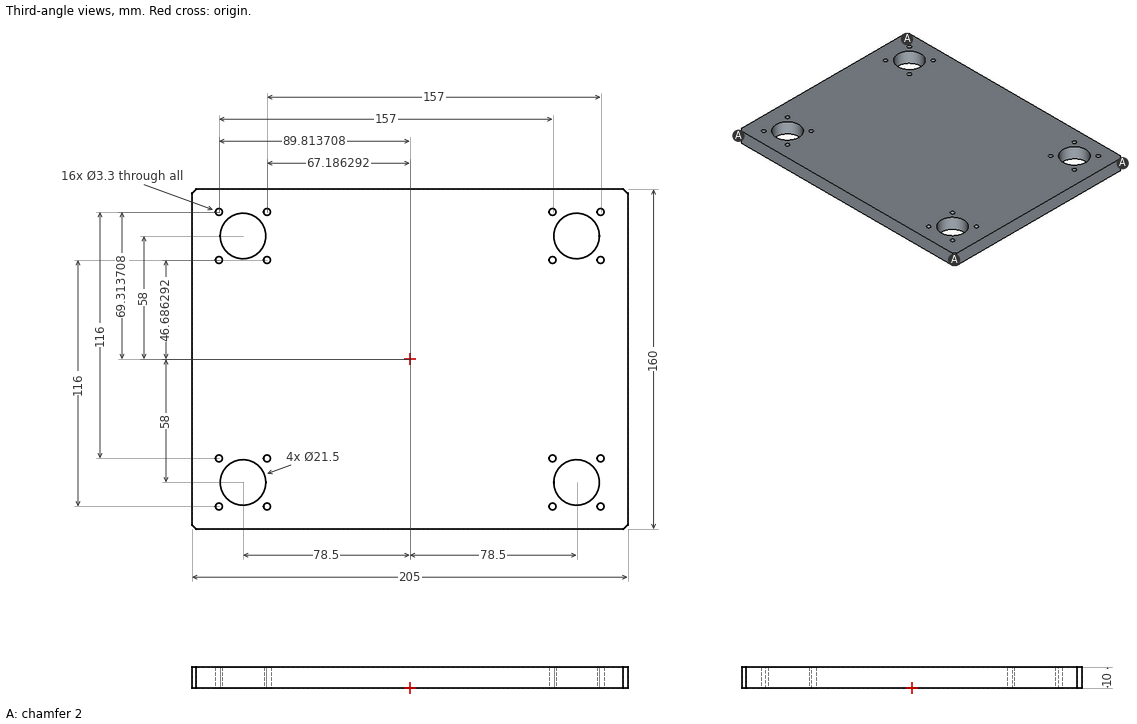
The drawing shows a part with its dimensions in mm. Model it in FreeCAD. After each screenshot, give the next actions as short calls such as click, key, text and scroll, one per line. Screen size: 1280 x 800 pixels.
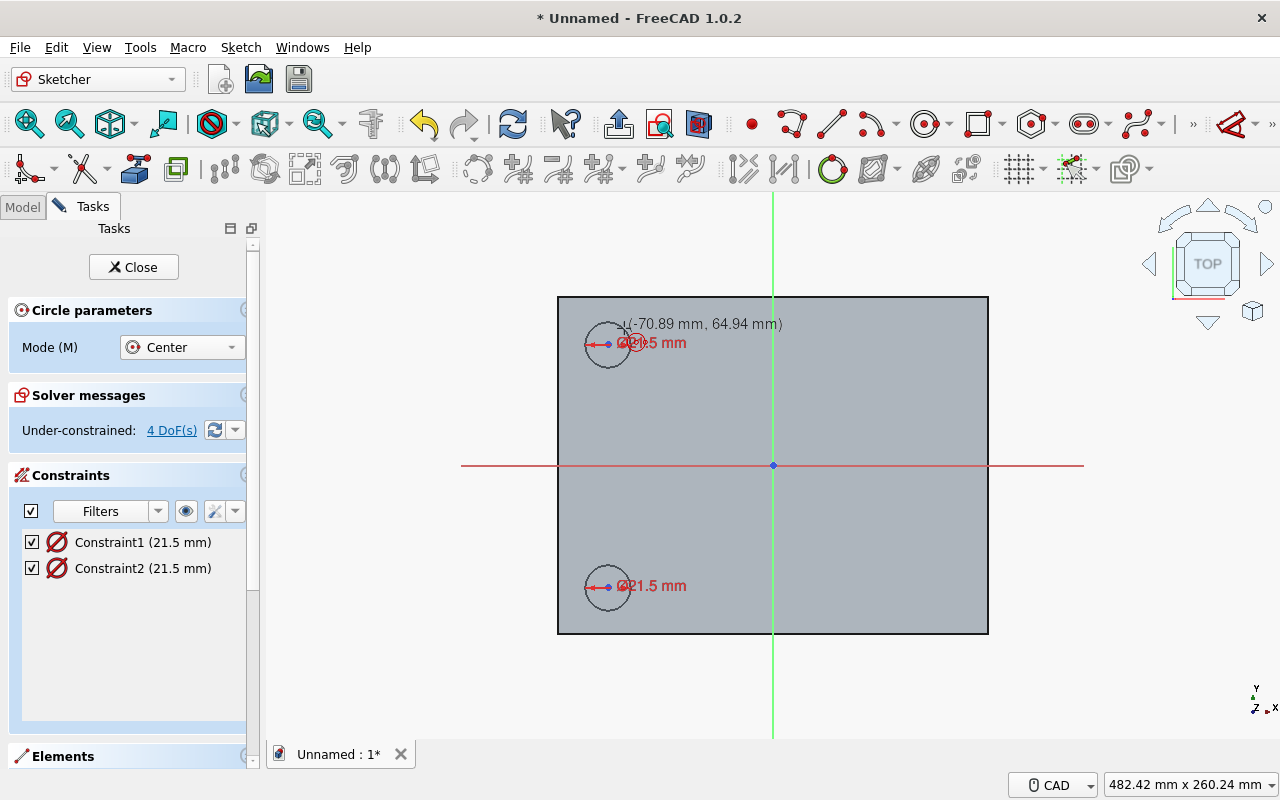
click(938, 587)
move(954, 571)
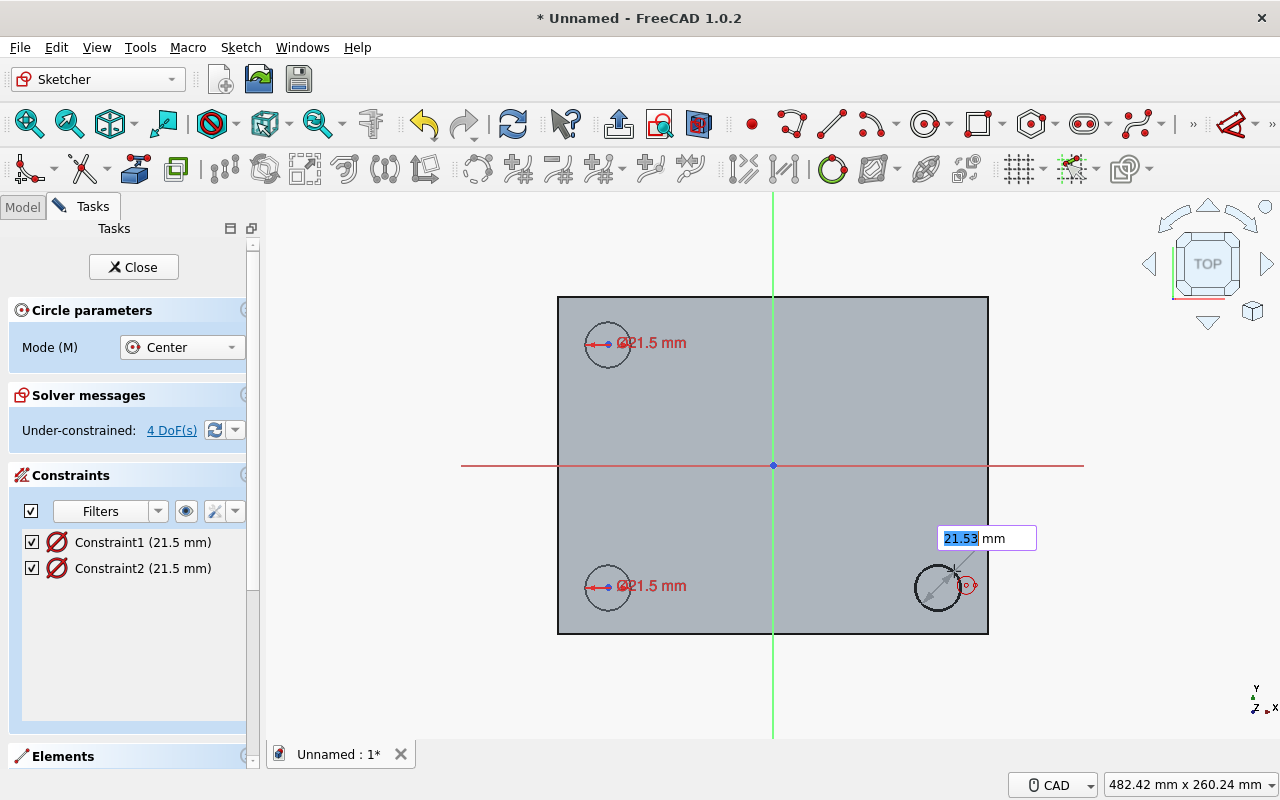
text(21.5)
key(Return)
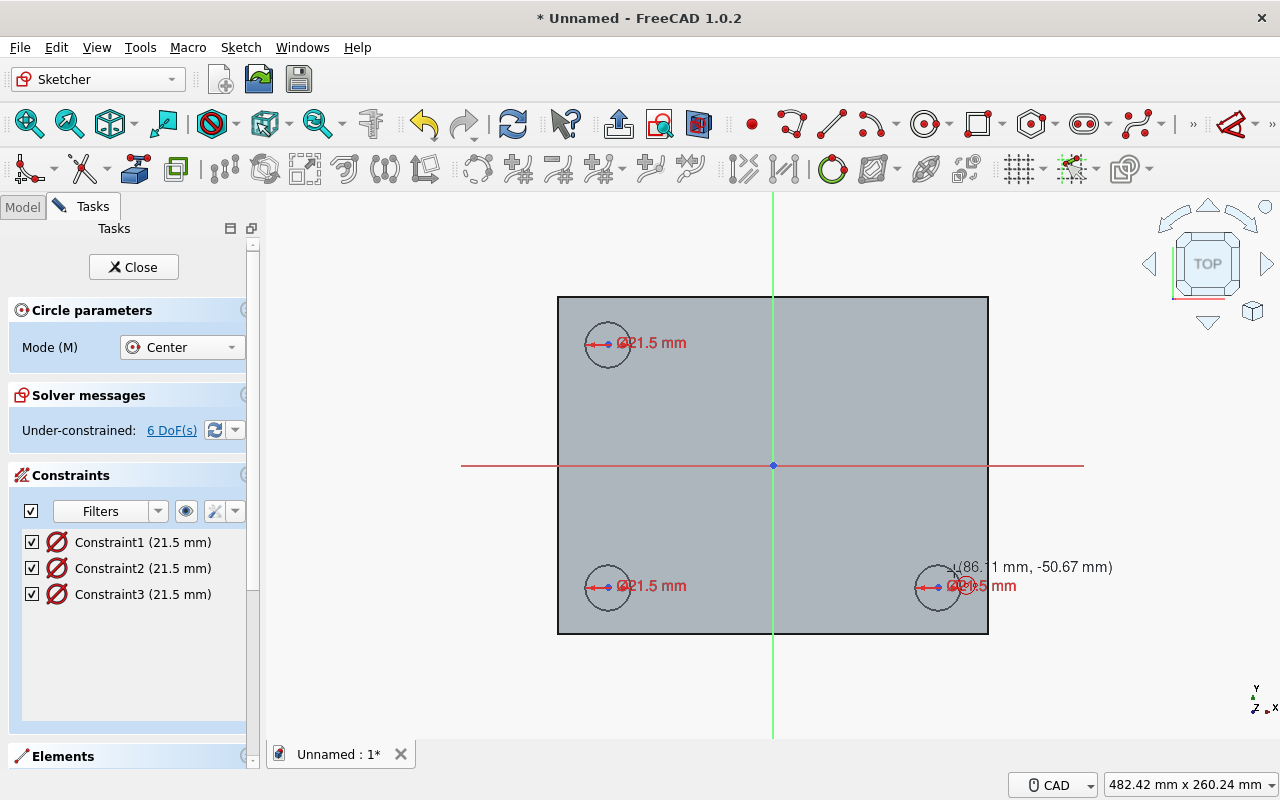
click(938, 344)
move(954, 328)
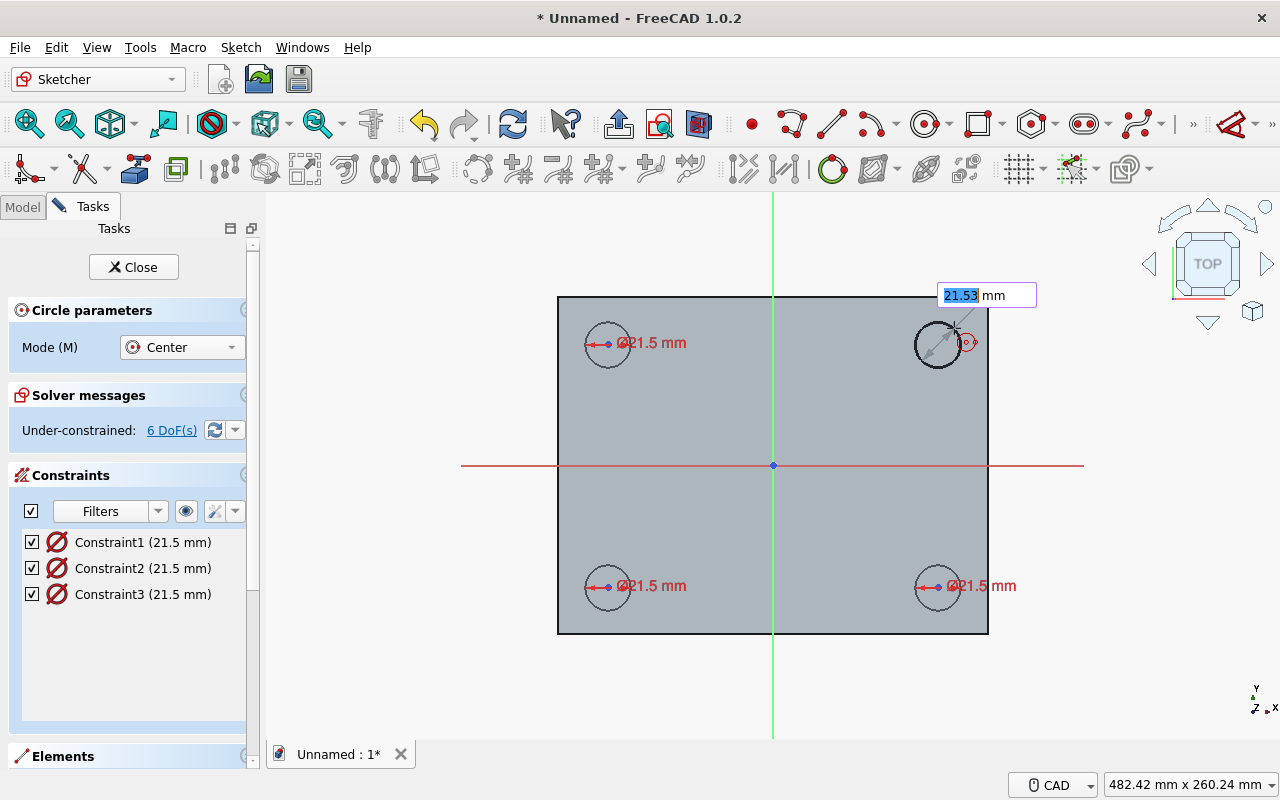
text(21.5)
key(Return)
key(Escape)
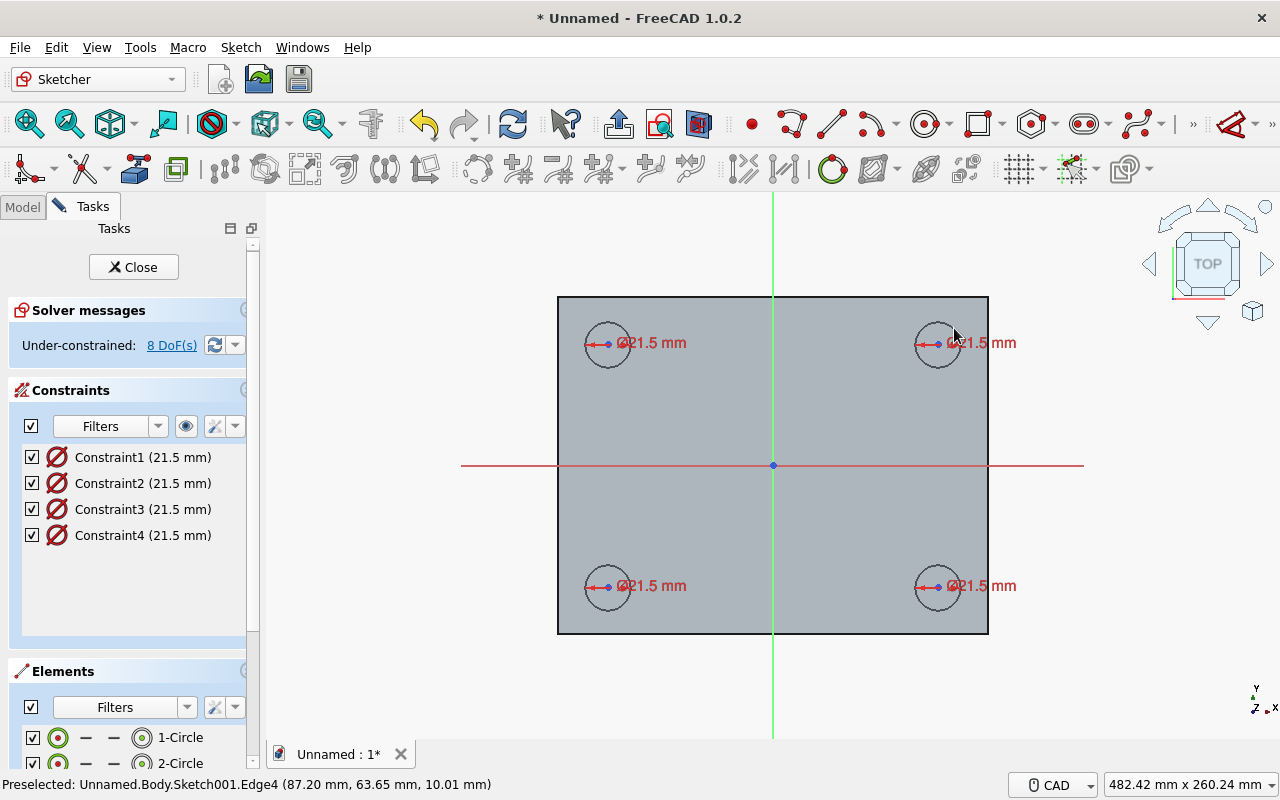
click(608, 588)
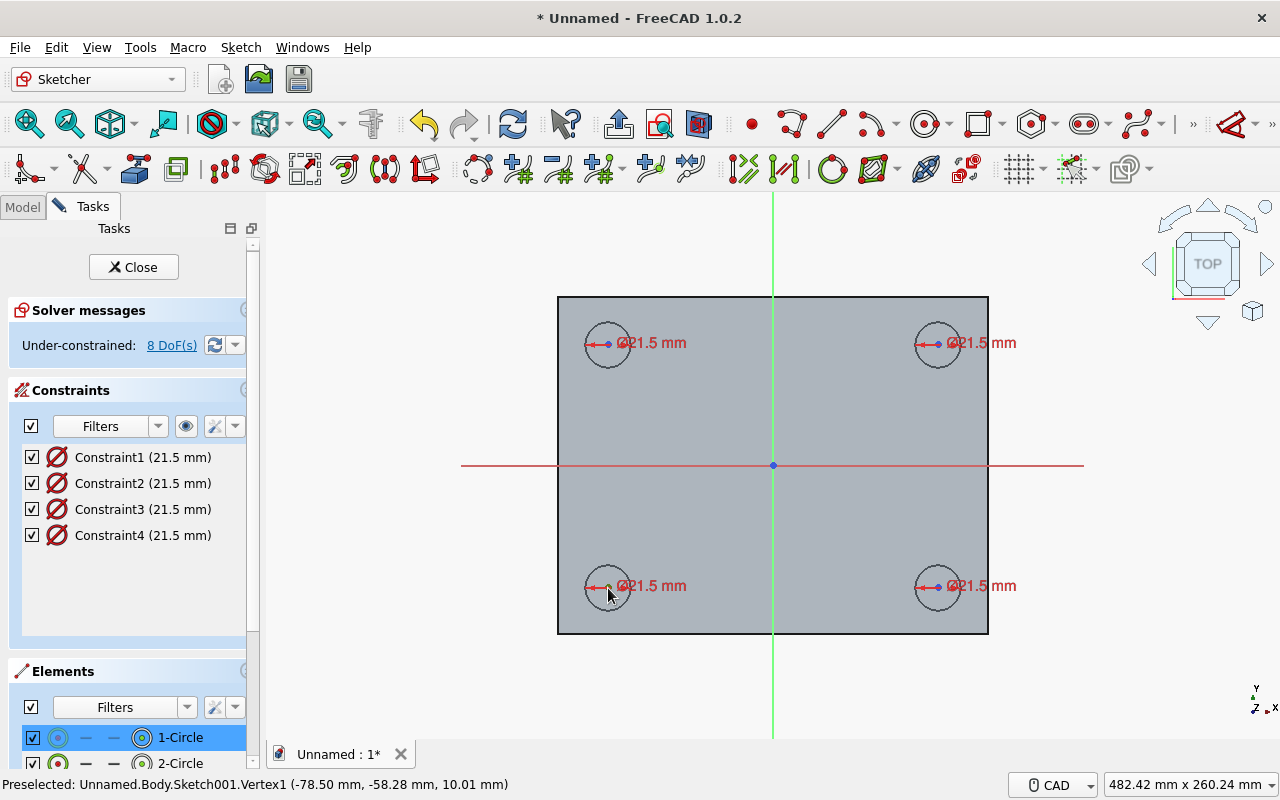
click(608, 345)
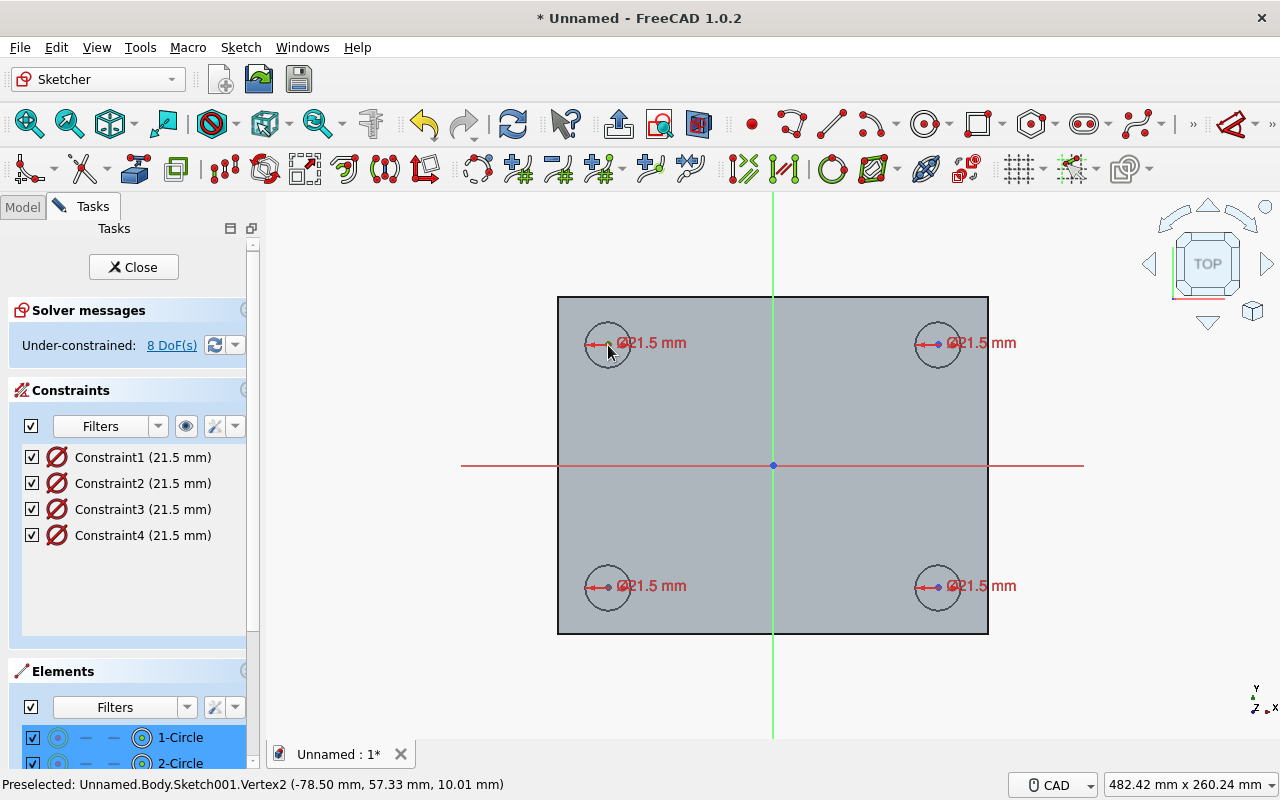
key(v)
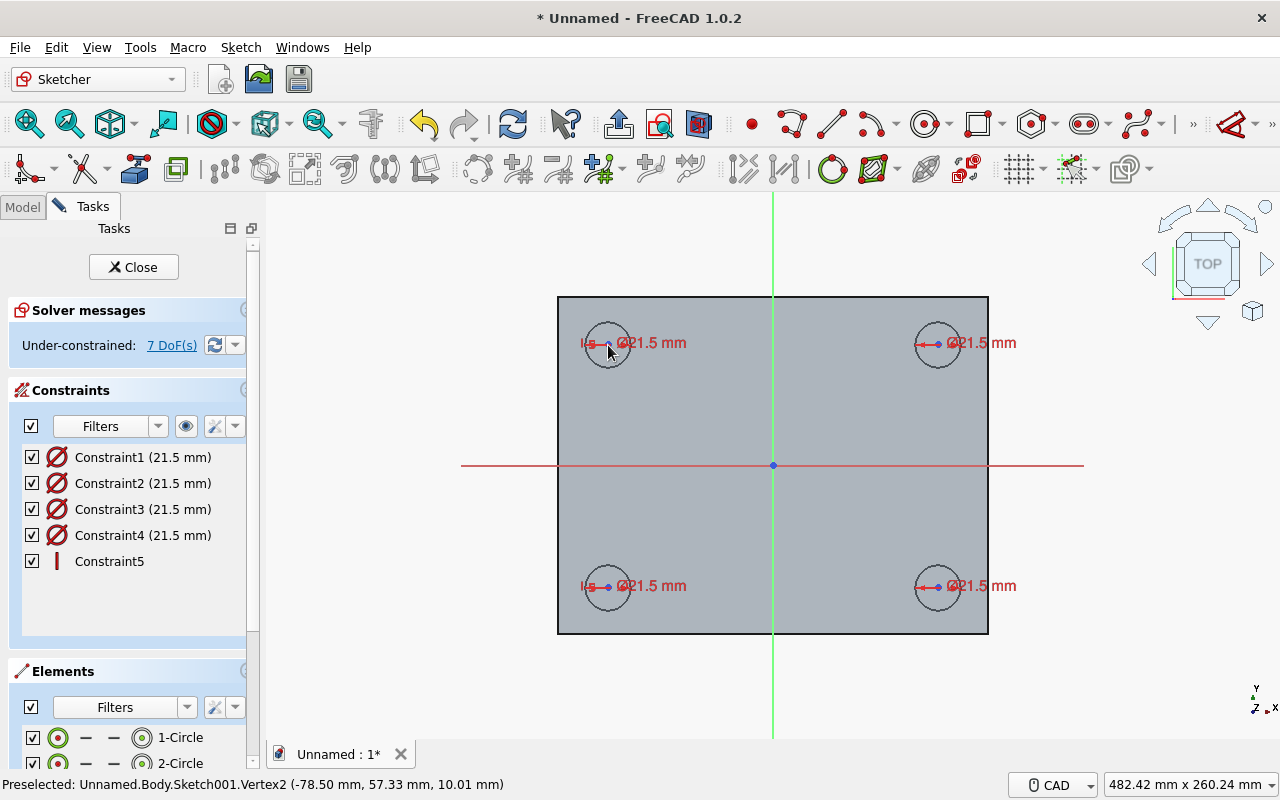
click(608, 588)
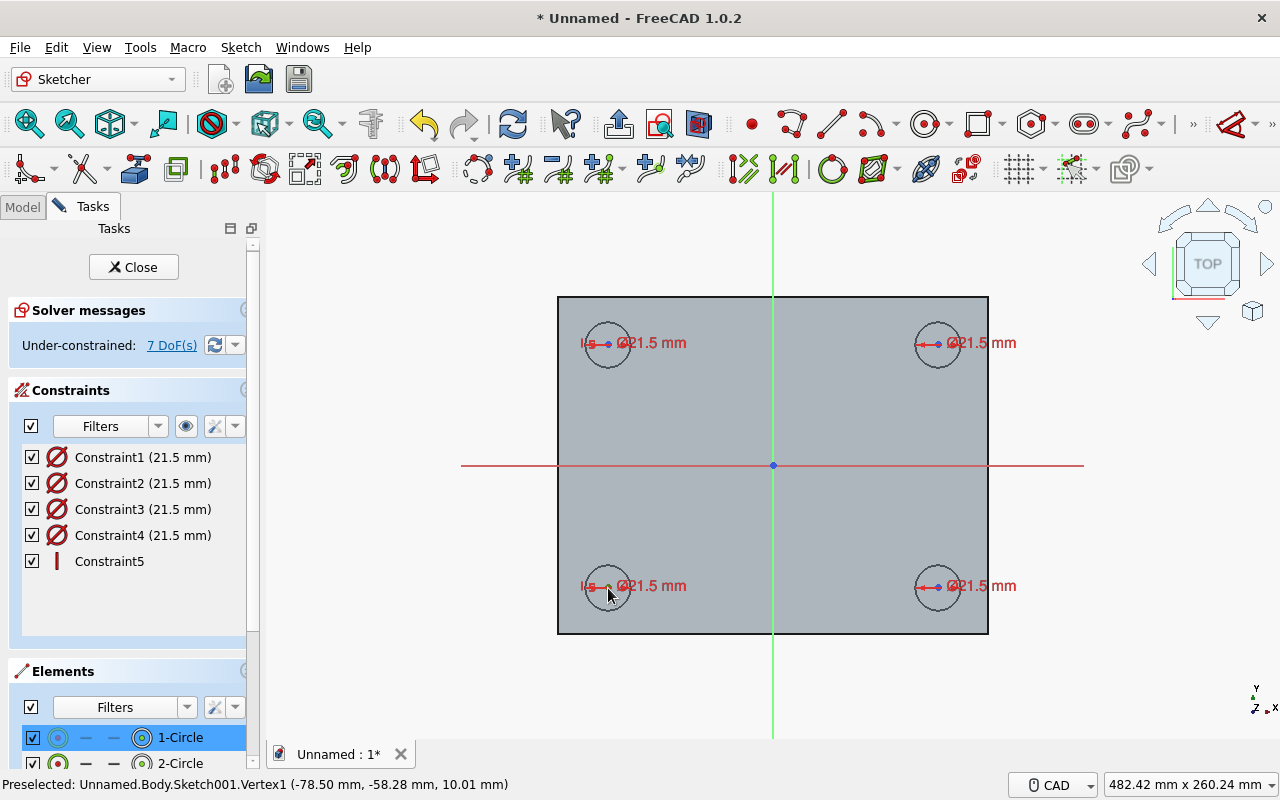
click(938, 588)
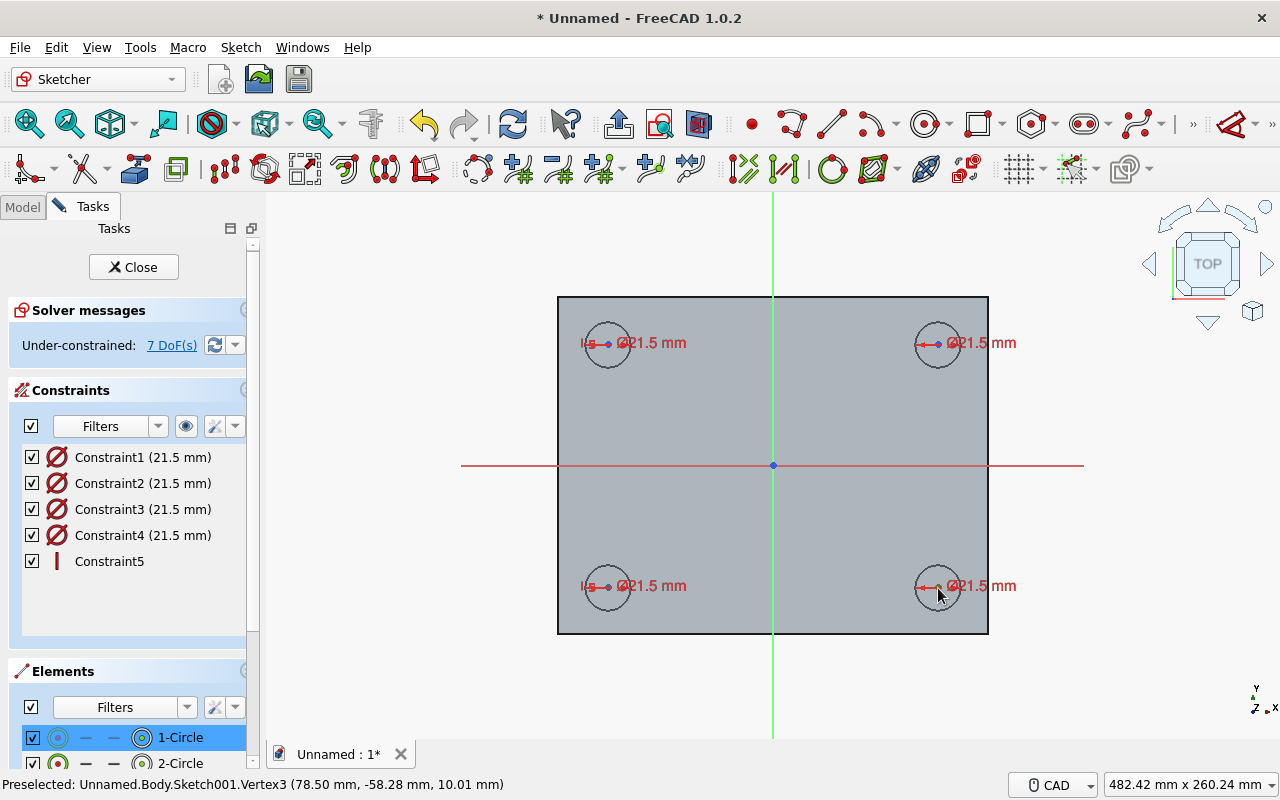
key(h)